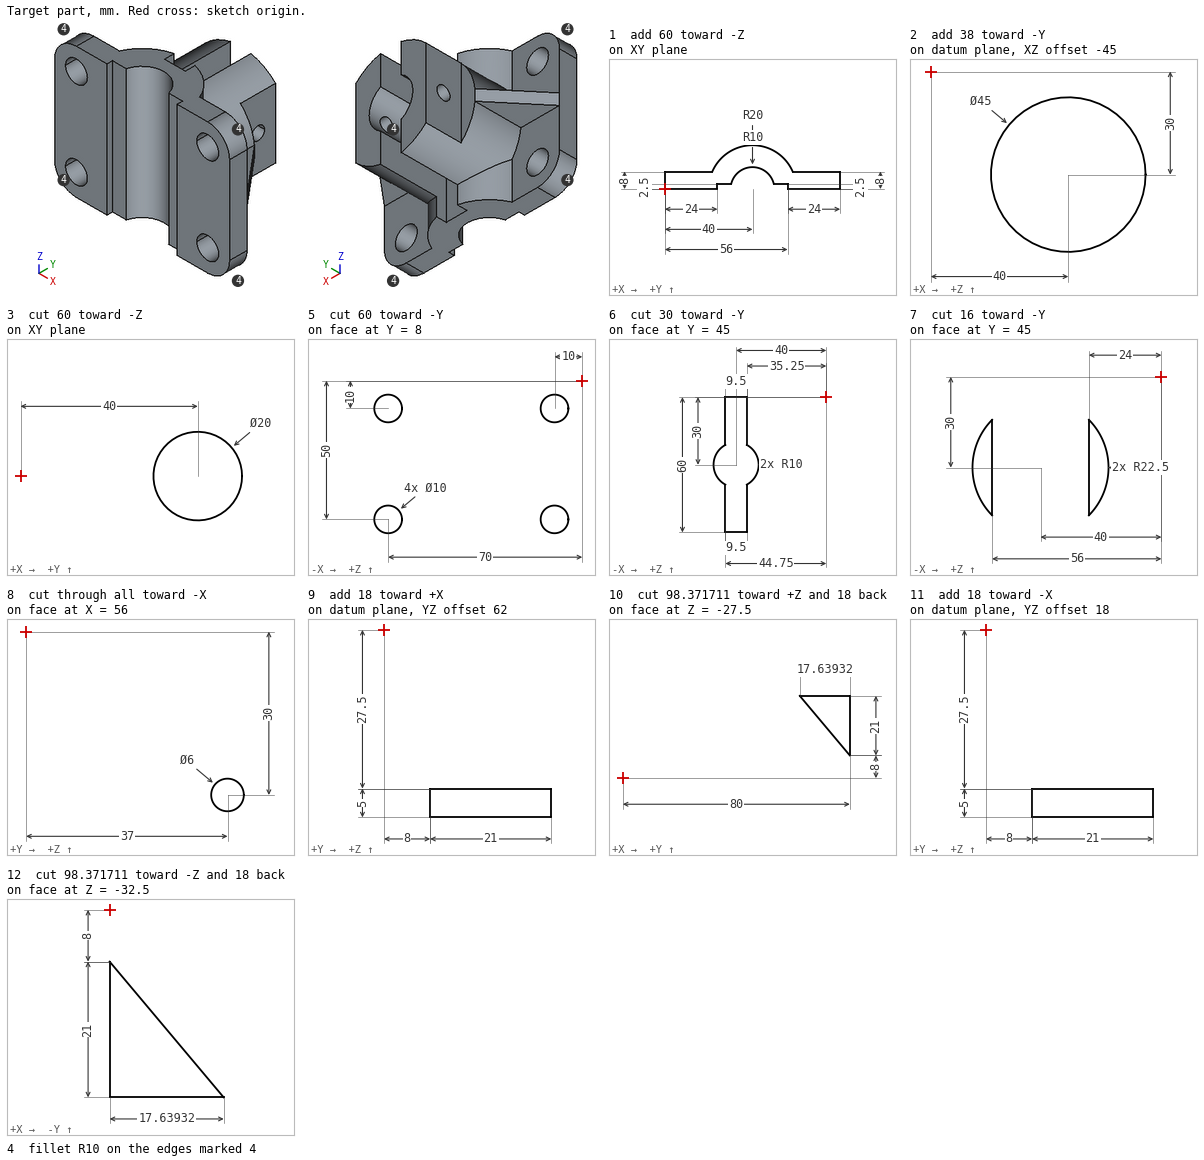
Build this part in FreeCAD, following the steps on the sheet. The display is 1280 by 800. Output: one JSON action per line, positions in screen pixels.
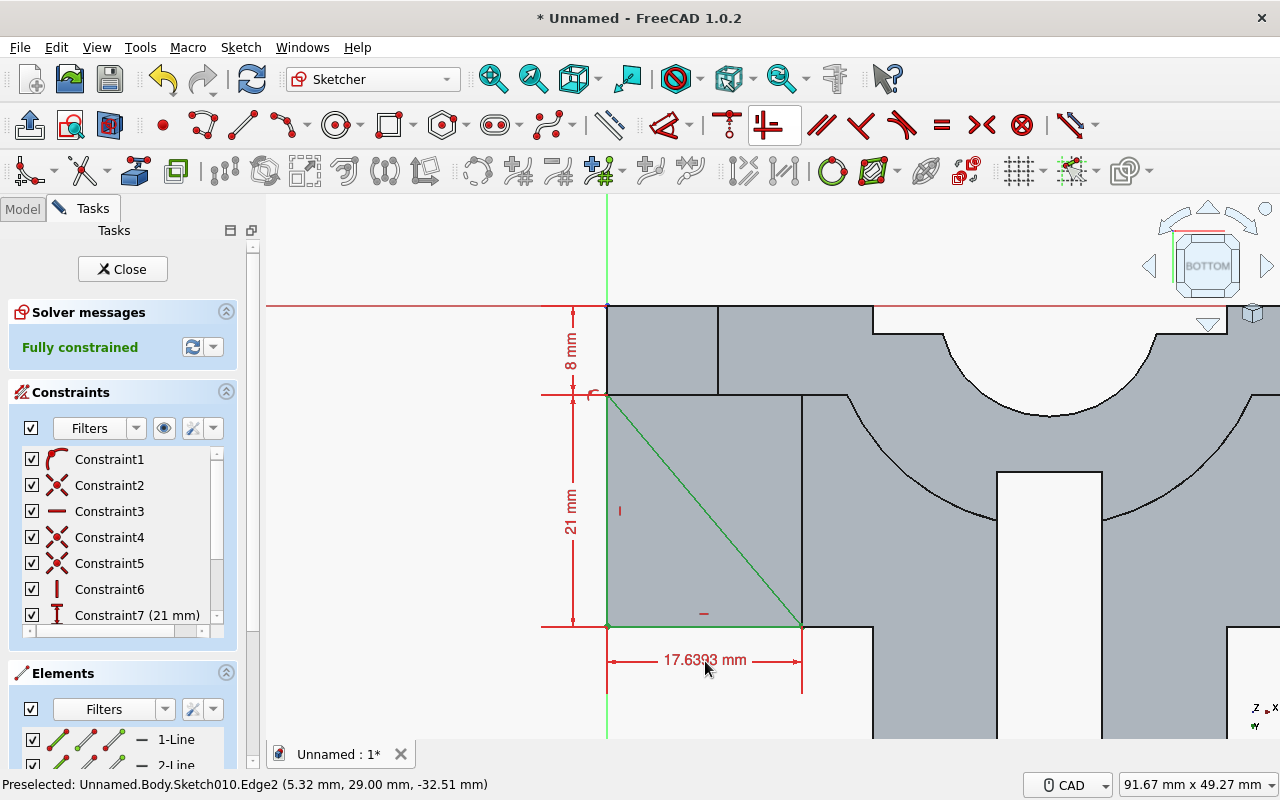
{"action": "left_click", "coordinate": [123, 269]}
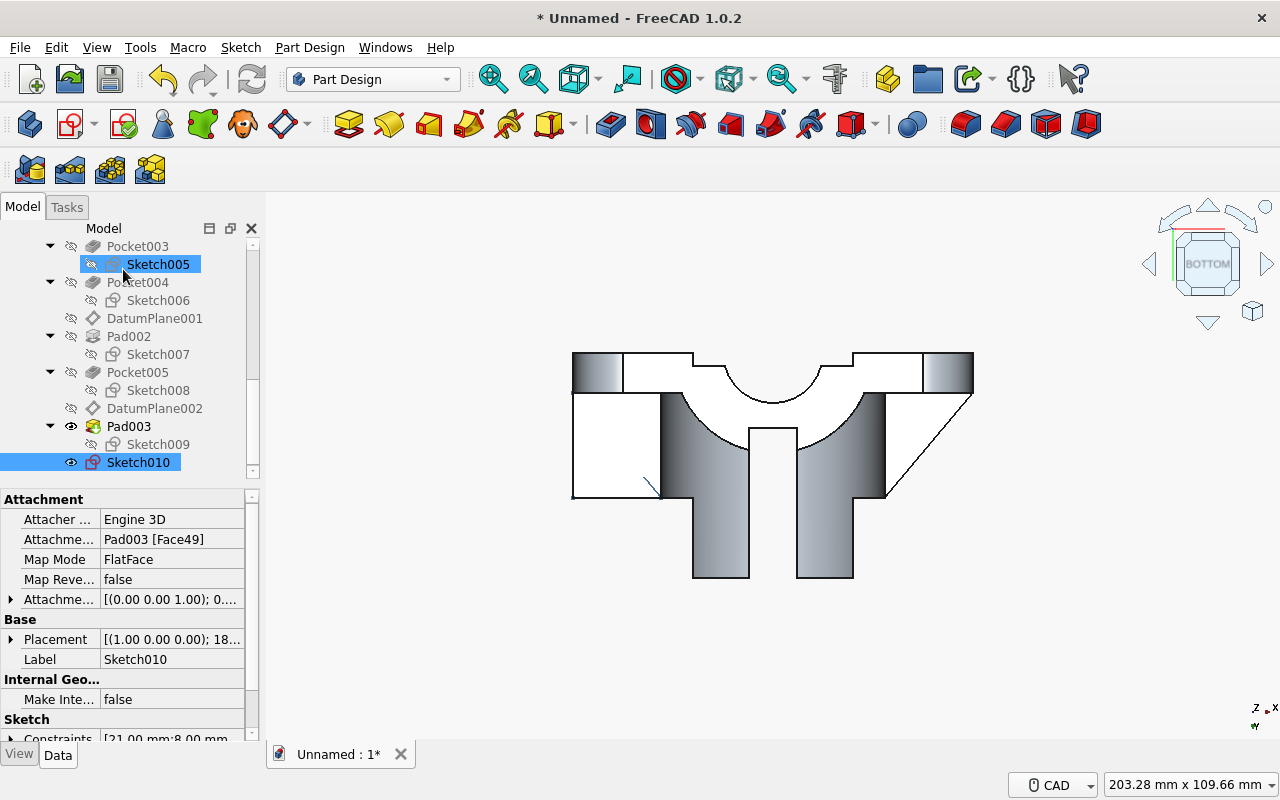
{"action": "left_click", "coordinate": [612, 124]}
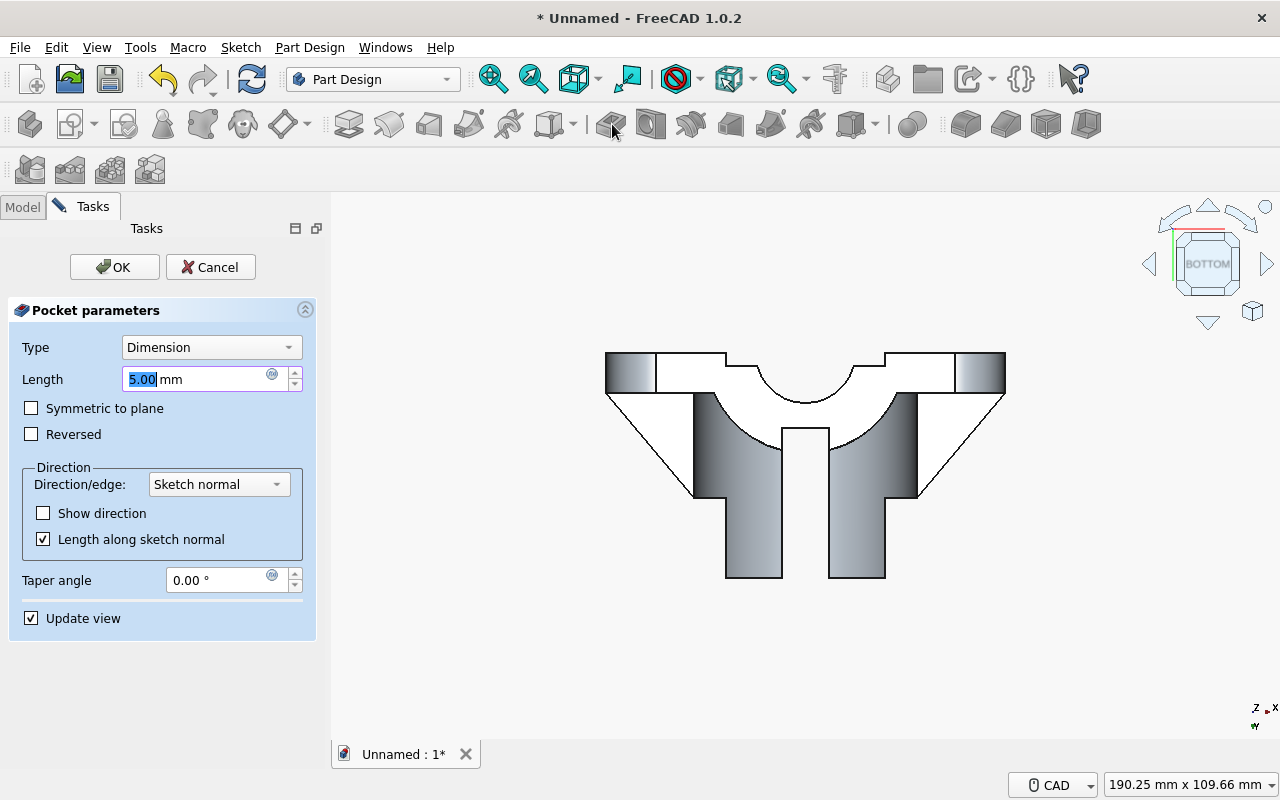
{"action": "left_click", "coordinate": [212, 348]}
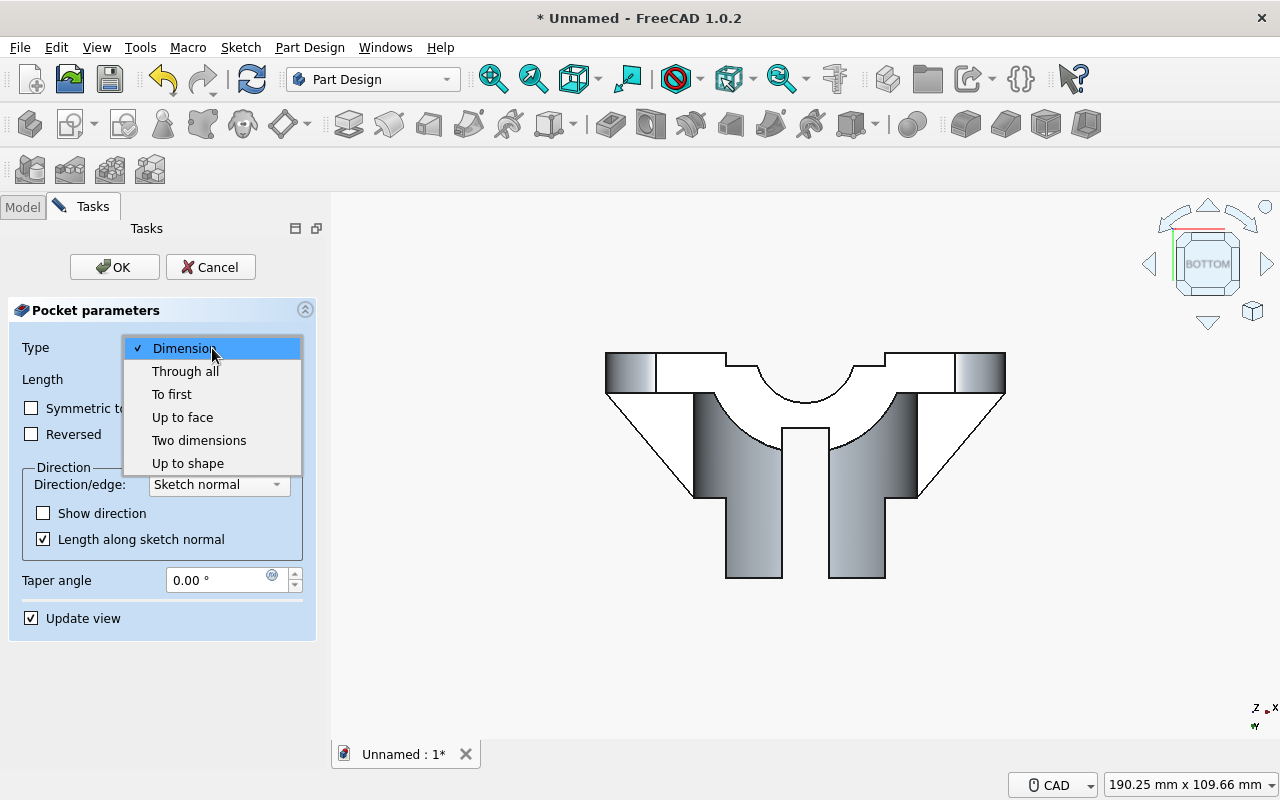
{"action": "left_click", "coordinate": [212, 440]}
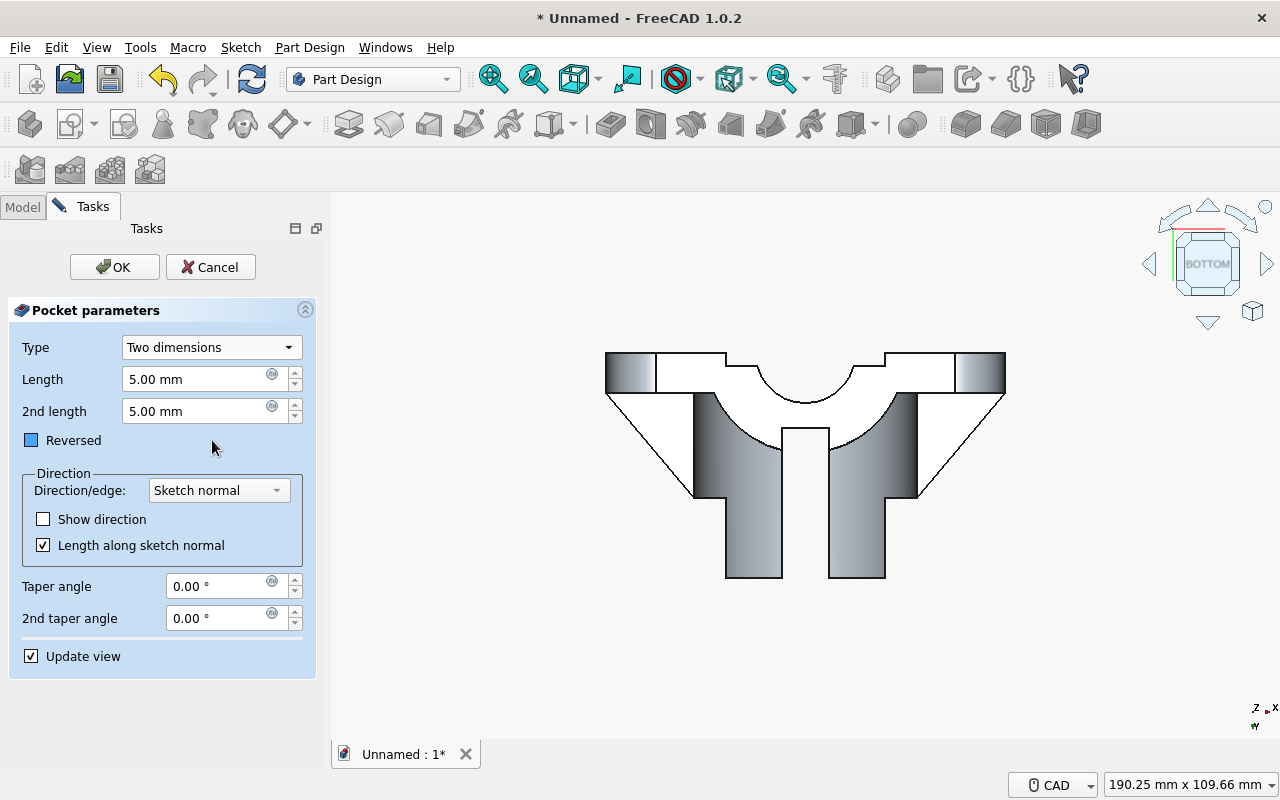
{"action": "triple_click", "coordinate": [204, 379]}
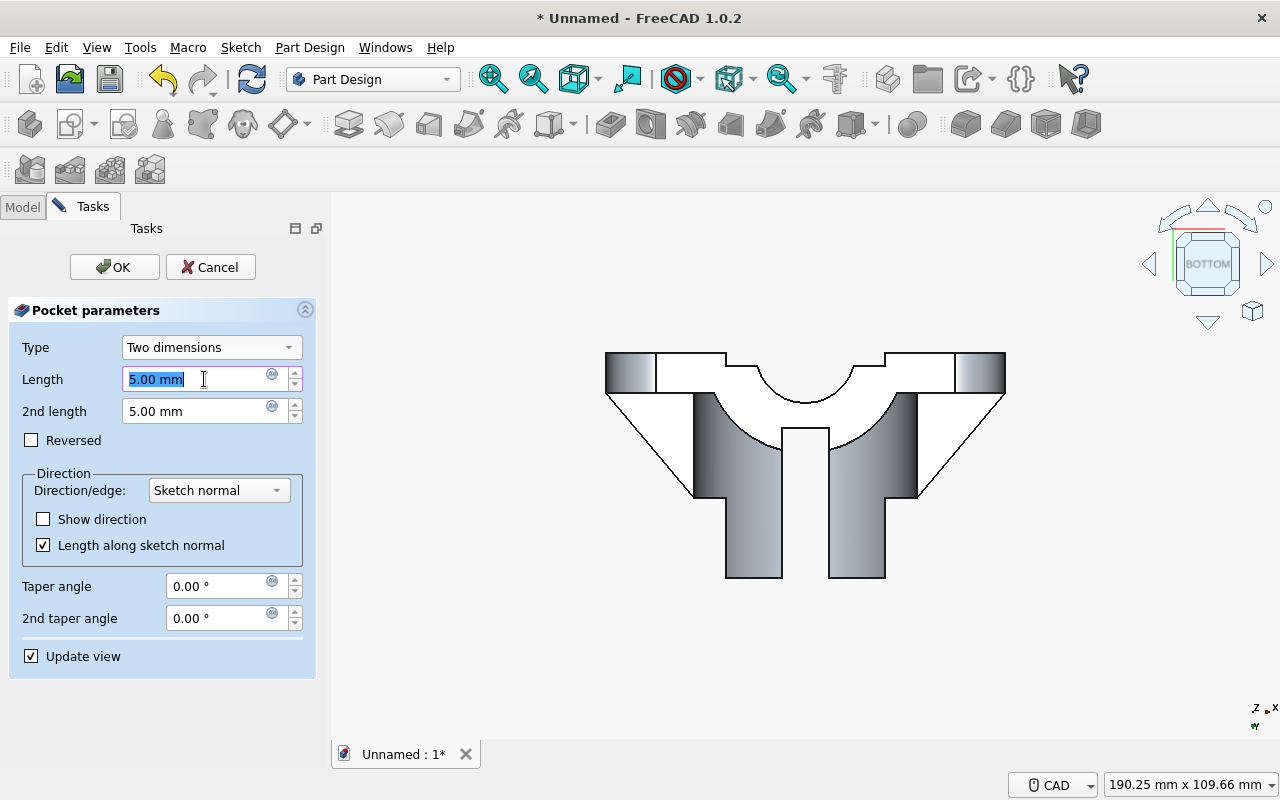
{"action": "type", "text": "98.371711"}
{"action": "key", "text": "Tab"}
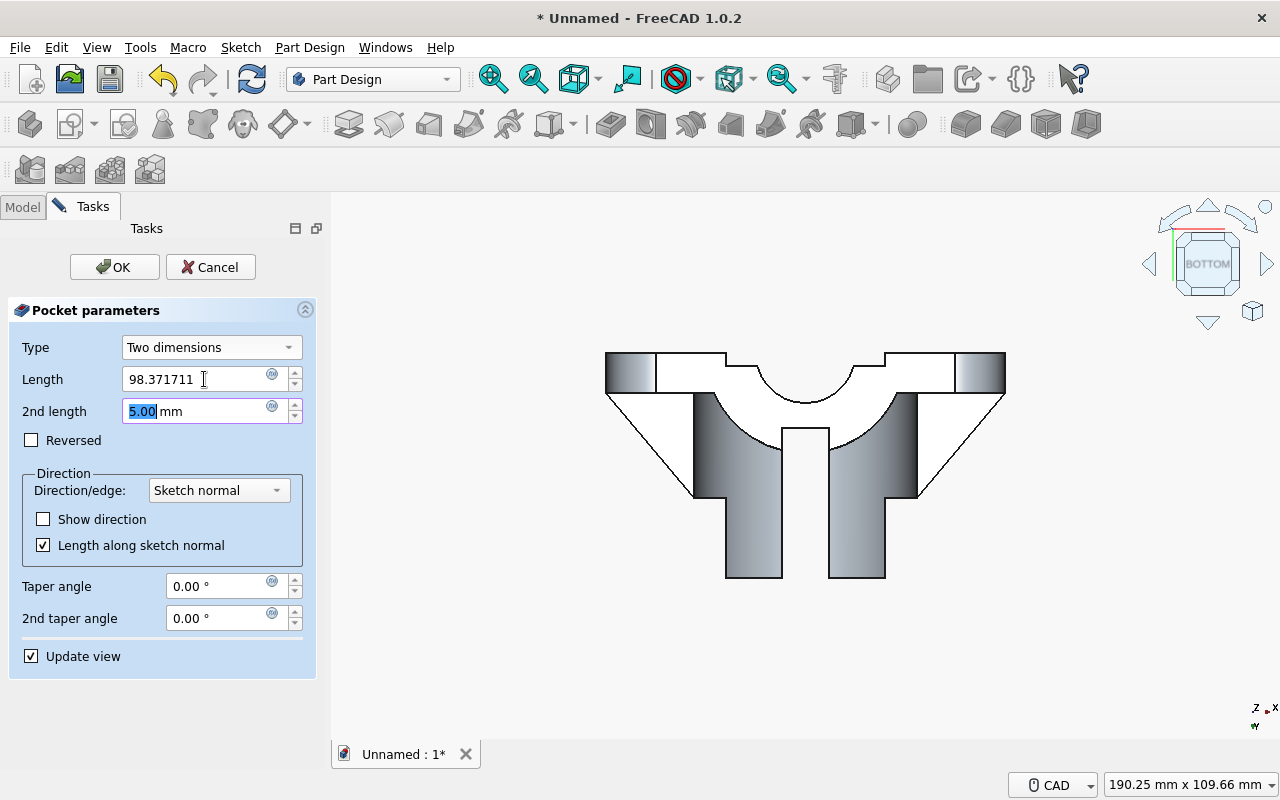
{"action": "type", "text": "18"}
{"action": "key", "text": "Tab"}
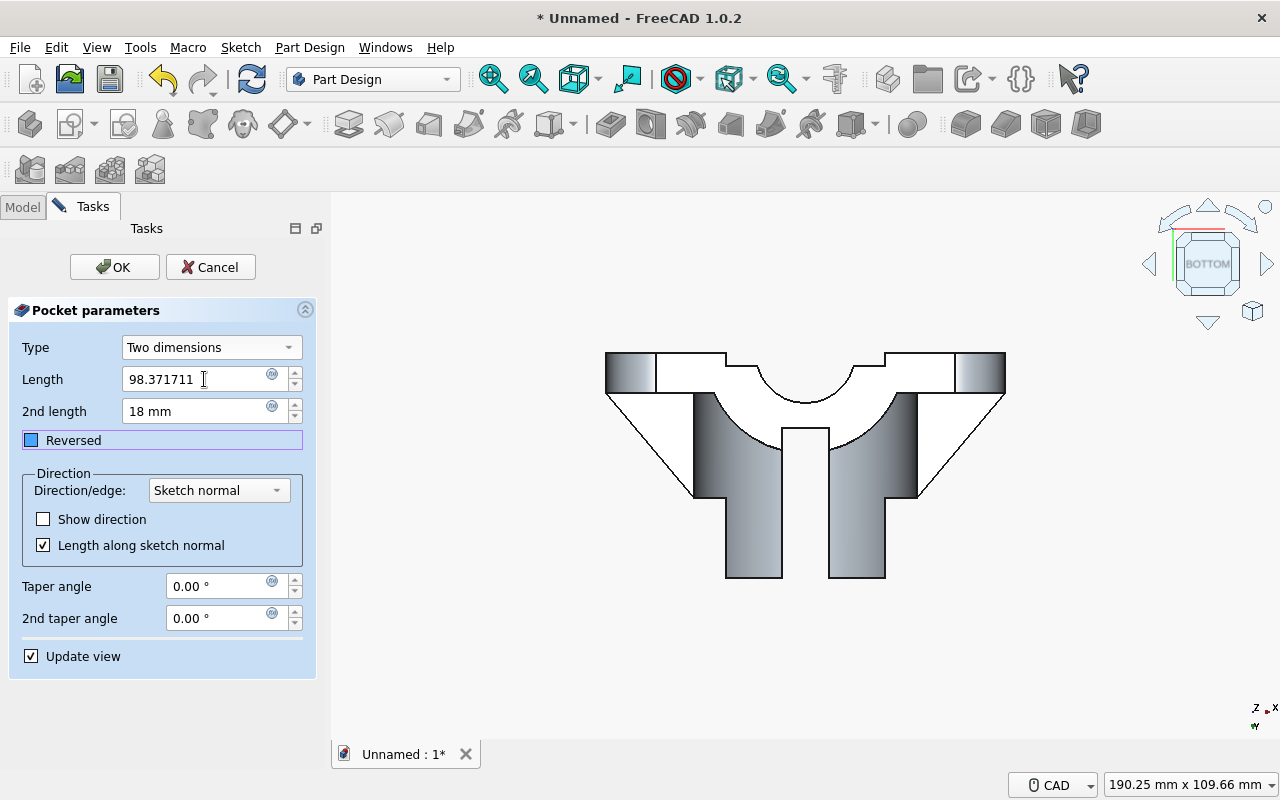
{"action": "left_click", "coordinate": [30, 440]}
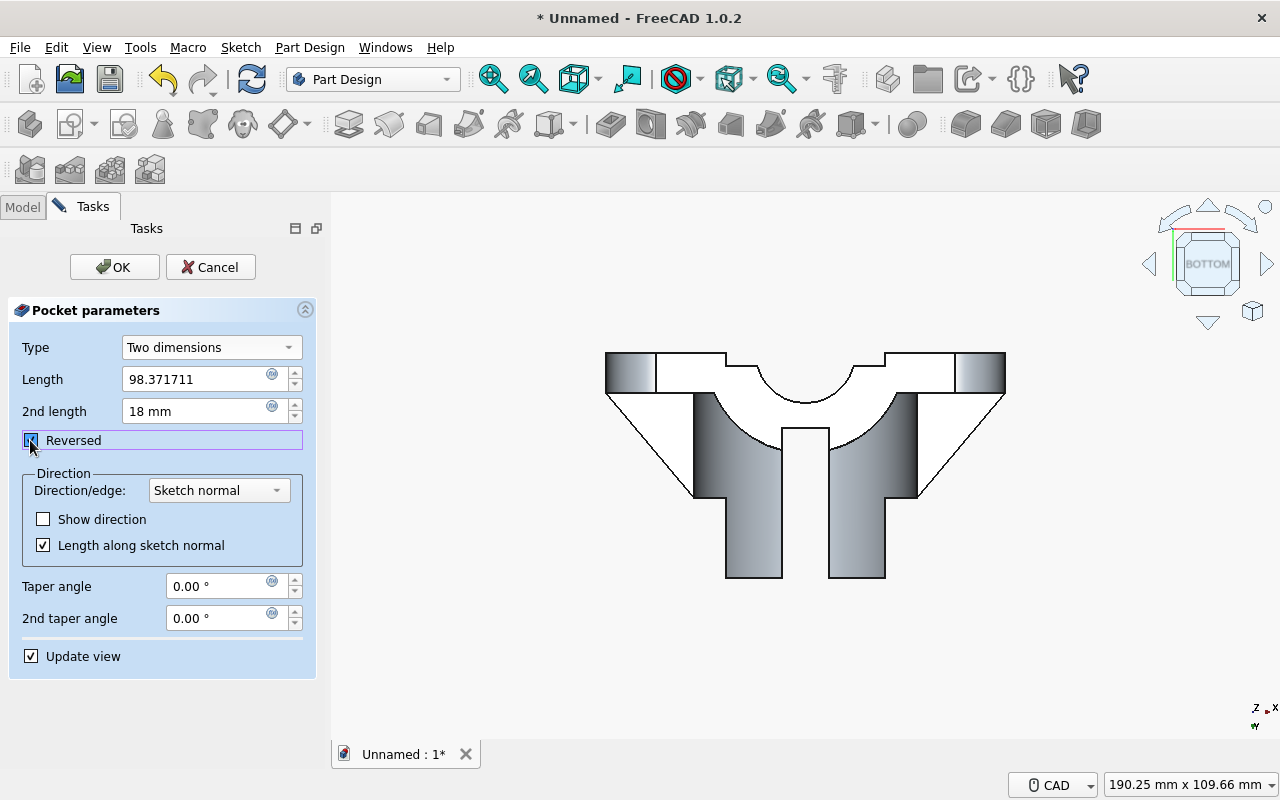
{"action": "left_click", "coordinate": [115, 267]}